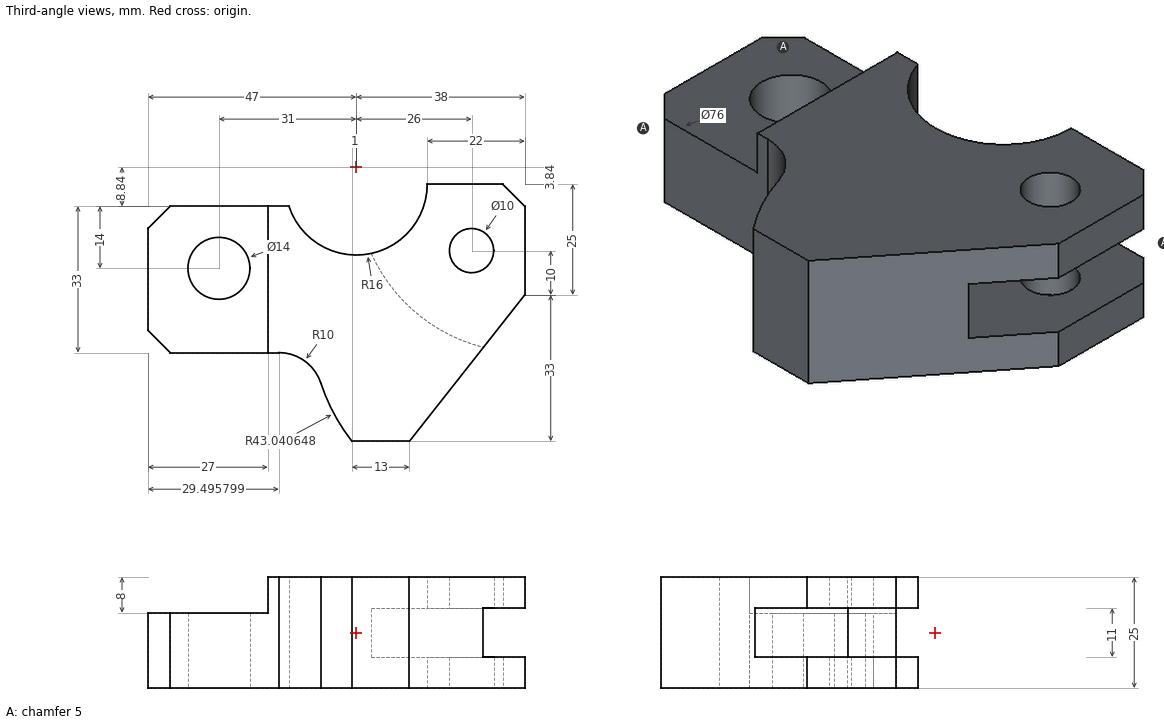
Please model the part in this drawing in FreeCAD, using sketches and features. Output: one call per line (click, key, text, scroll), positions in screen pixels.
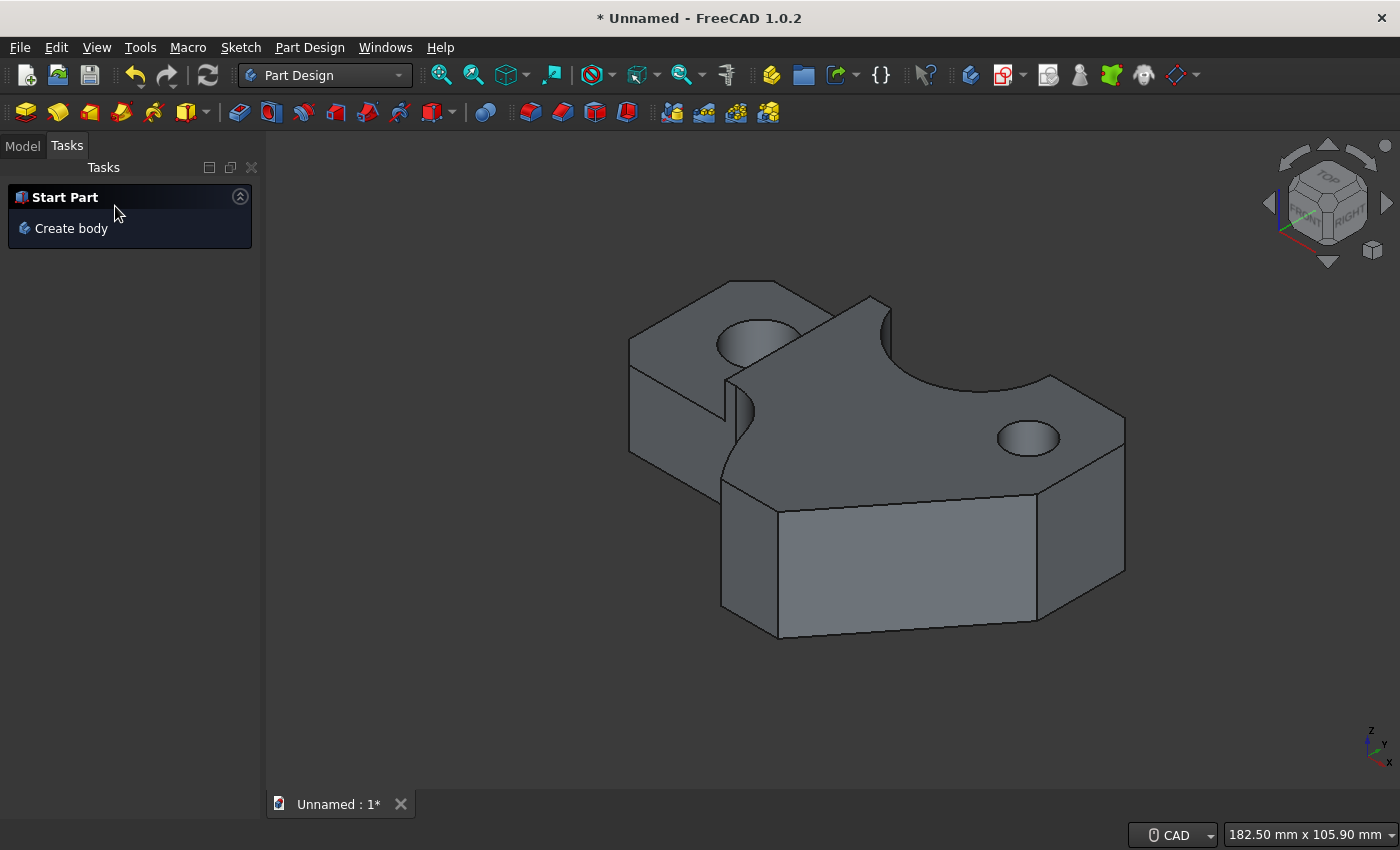
click(1004, 76)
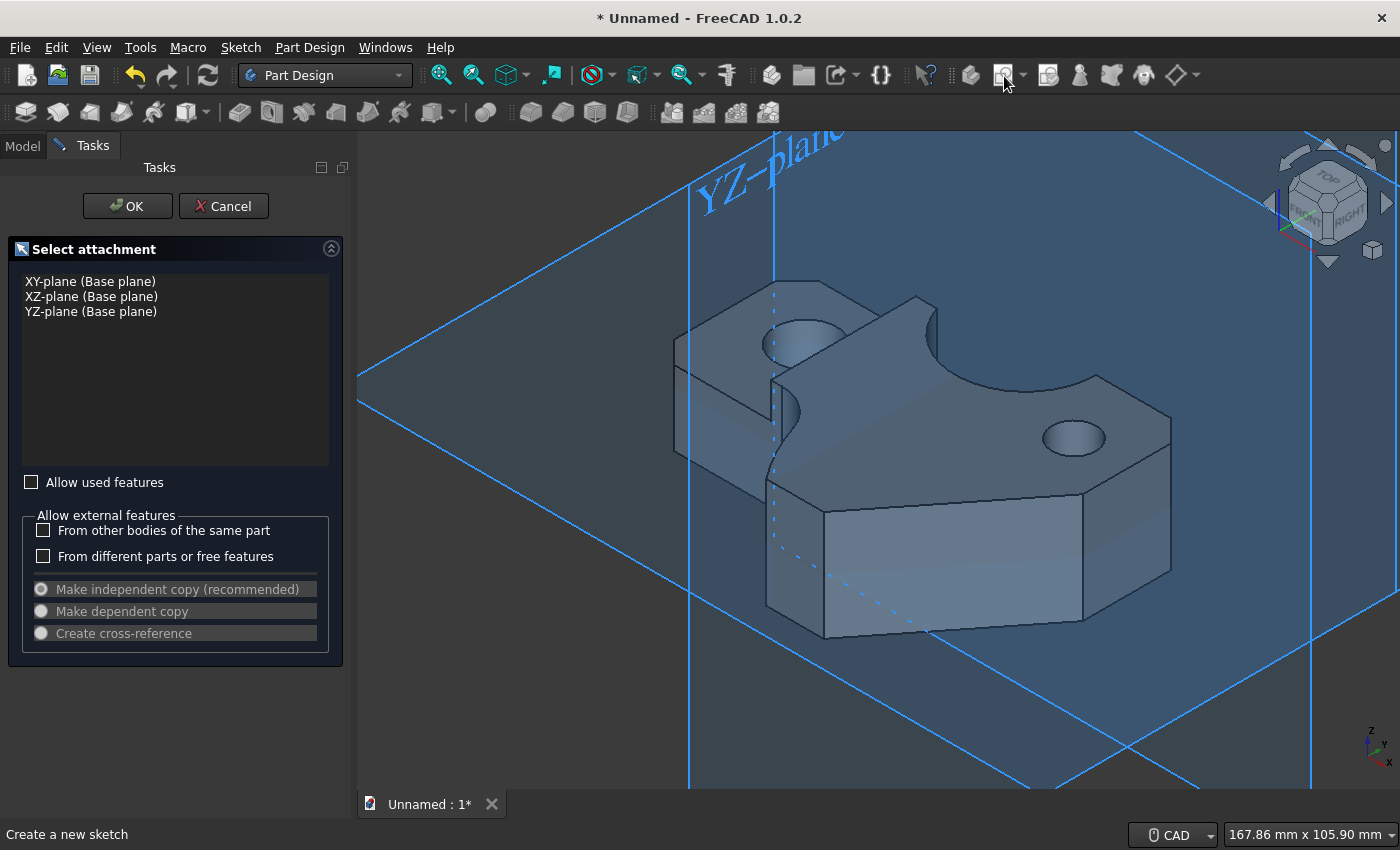
click(82, 282)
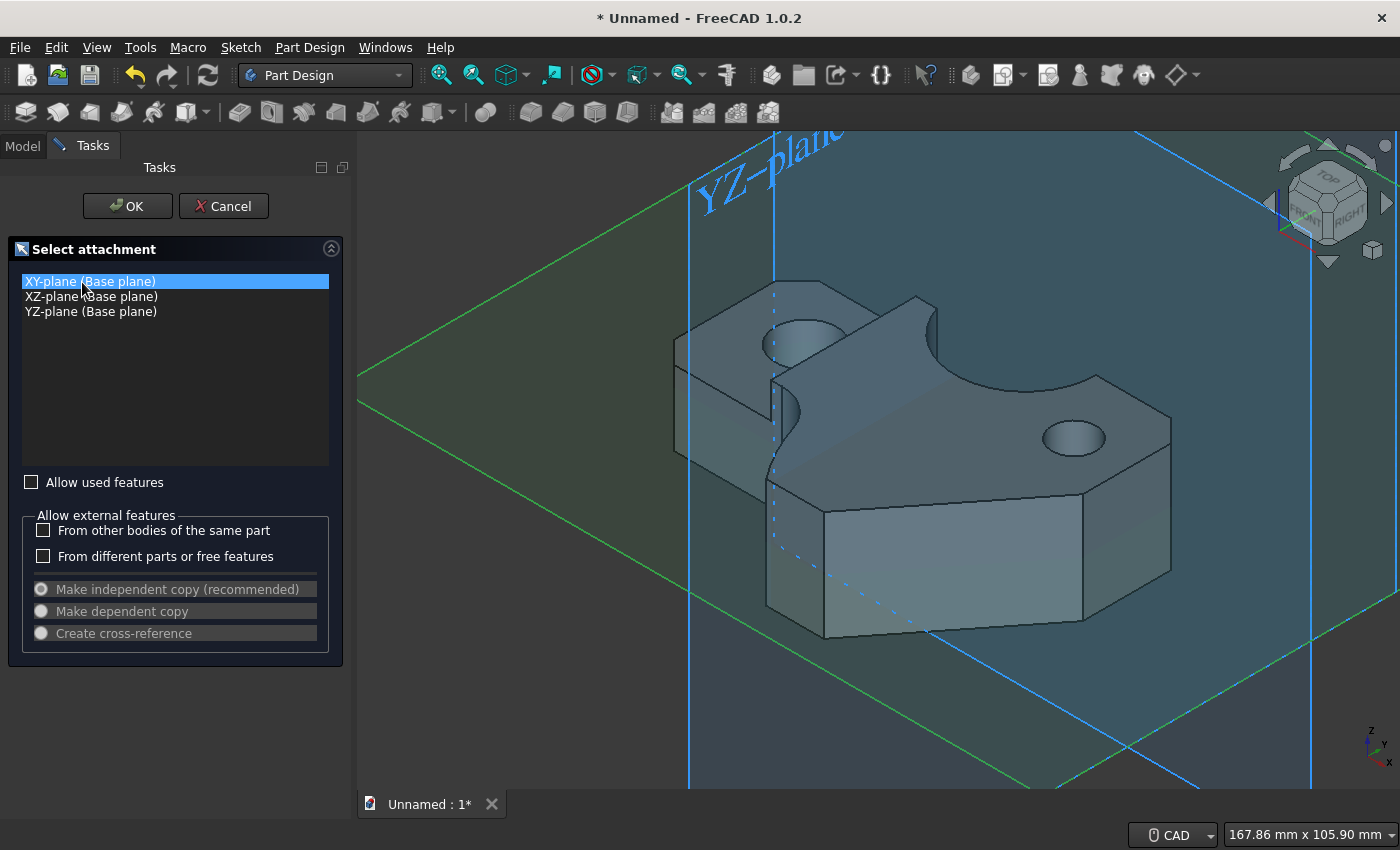
click(128, 206)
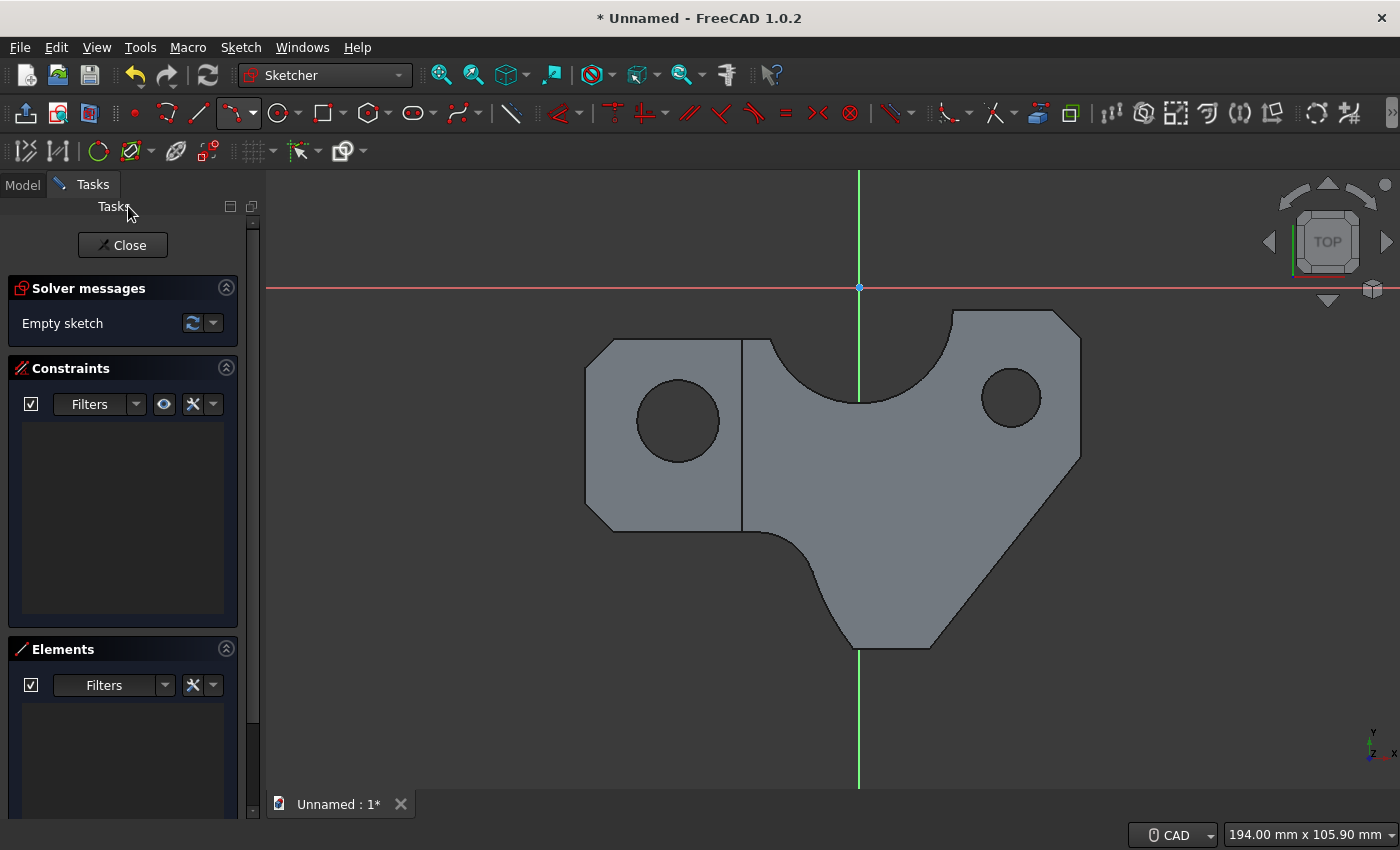
key(q)
key(s)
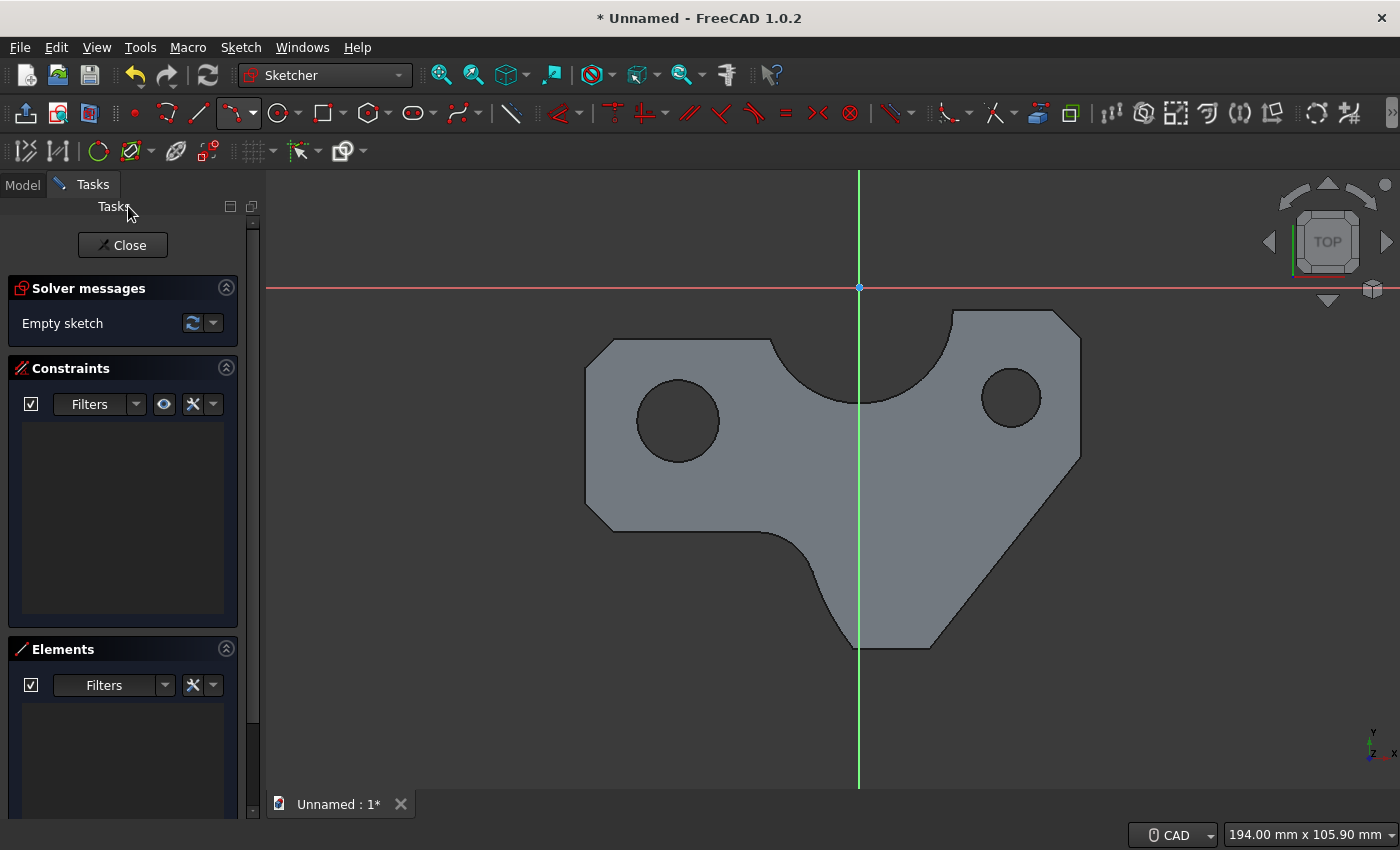
scroll(294, 761, down, 2)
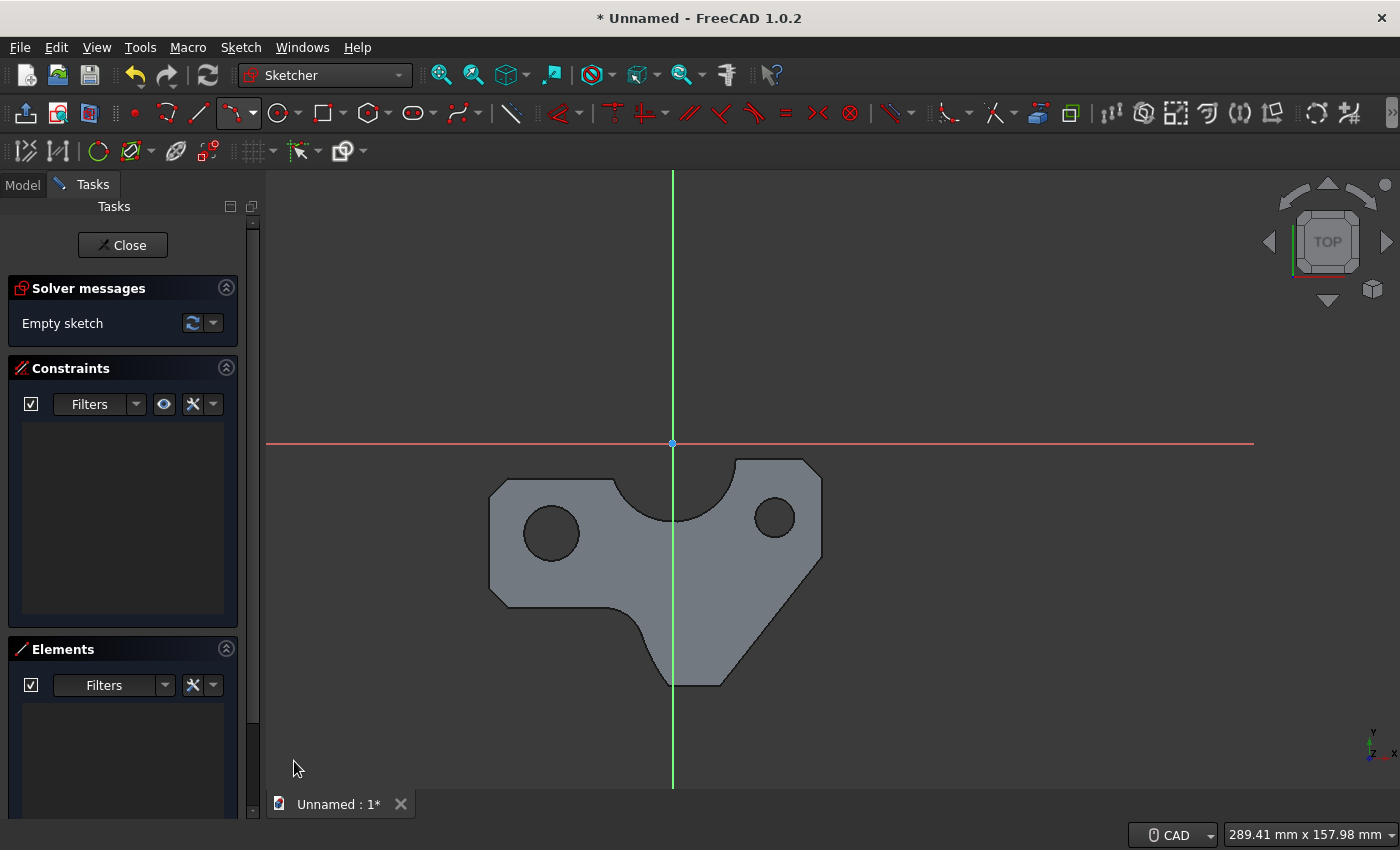
key(g)
key(c)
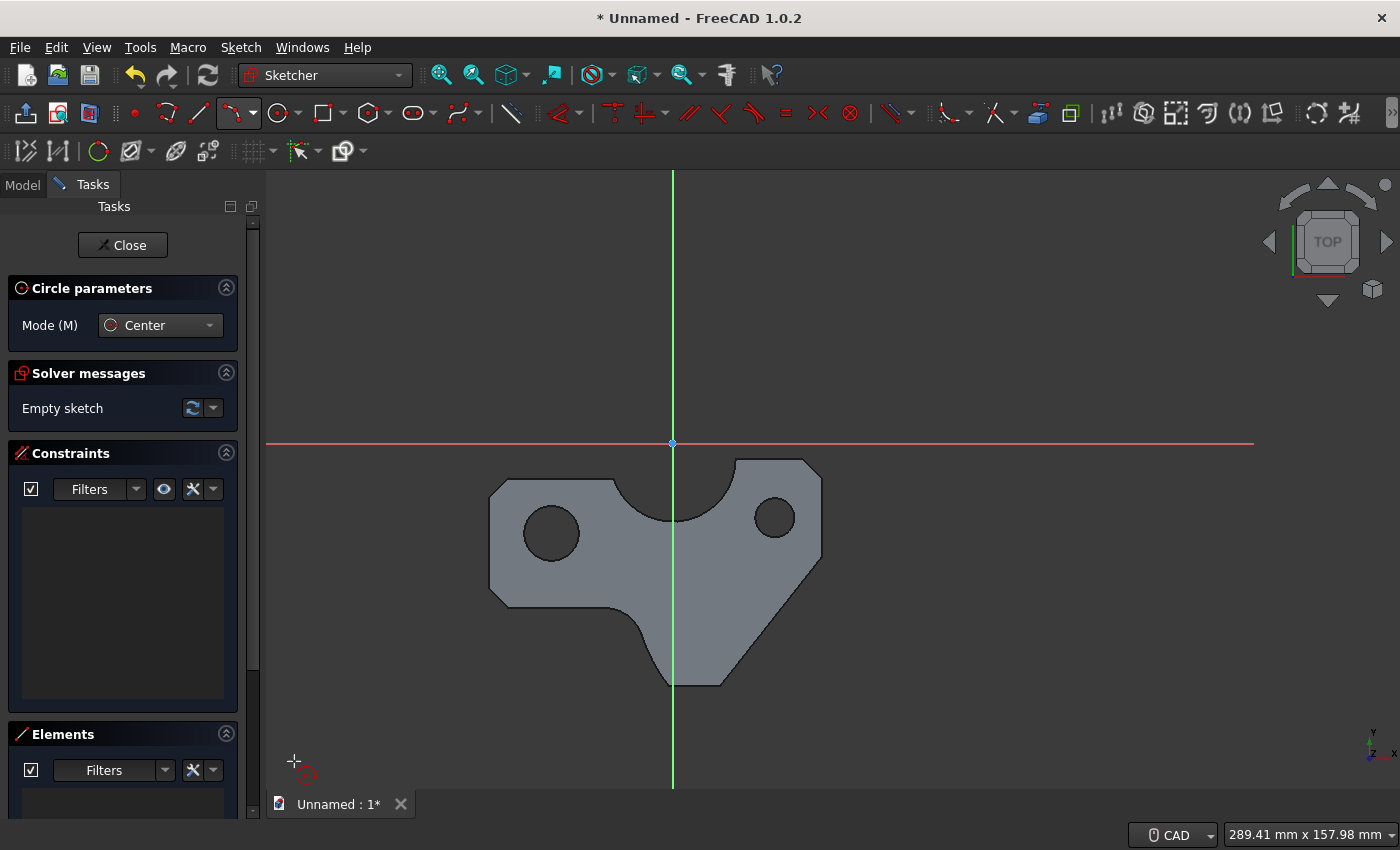
click(822, 459)
move(927, 354)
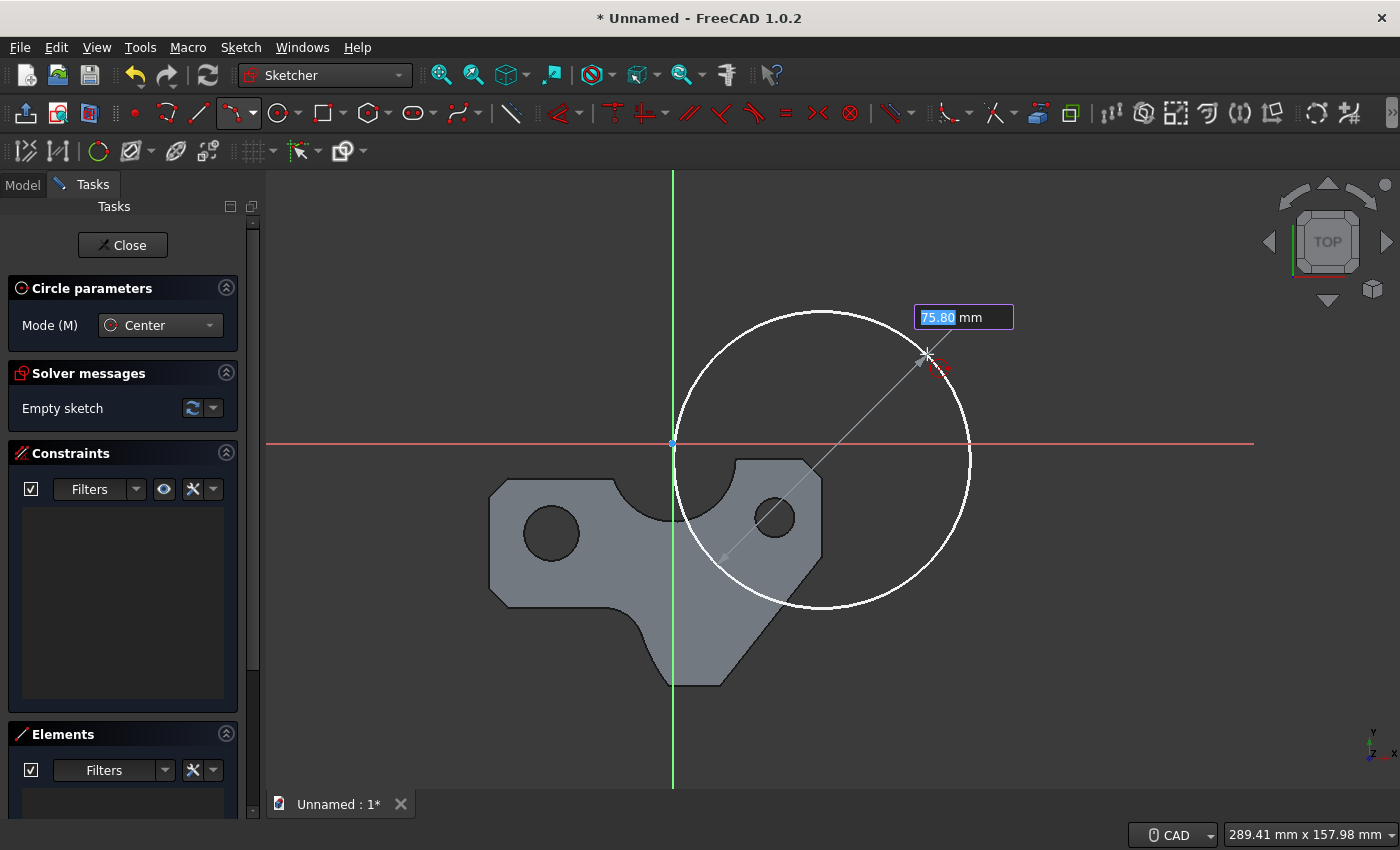
text(76)
key(Return)
key(Escape)